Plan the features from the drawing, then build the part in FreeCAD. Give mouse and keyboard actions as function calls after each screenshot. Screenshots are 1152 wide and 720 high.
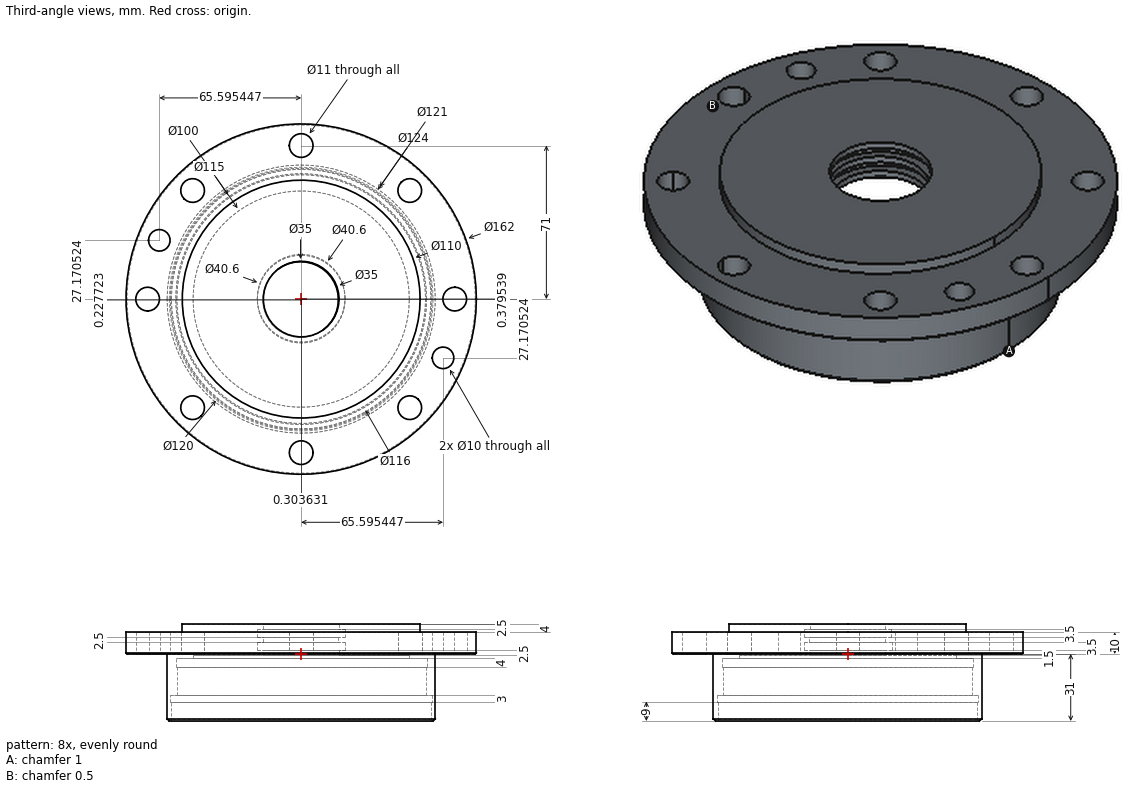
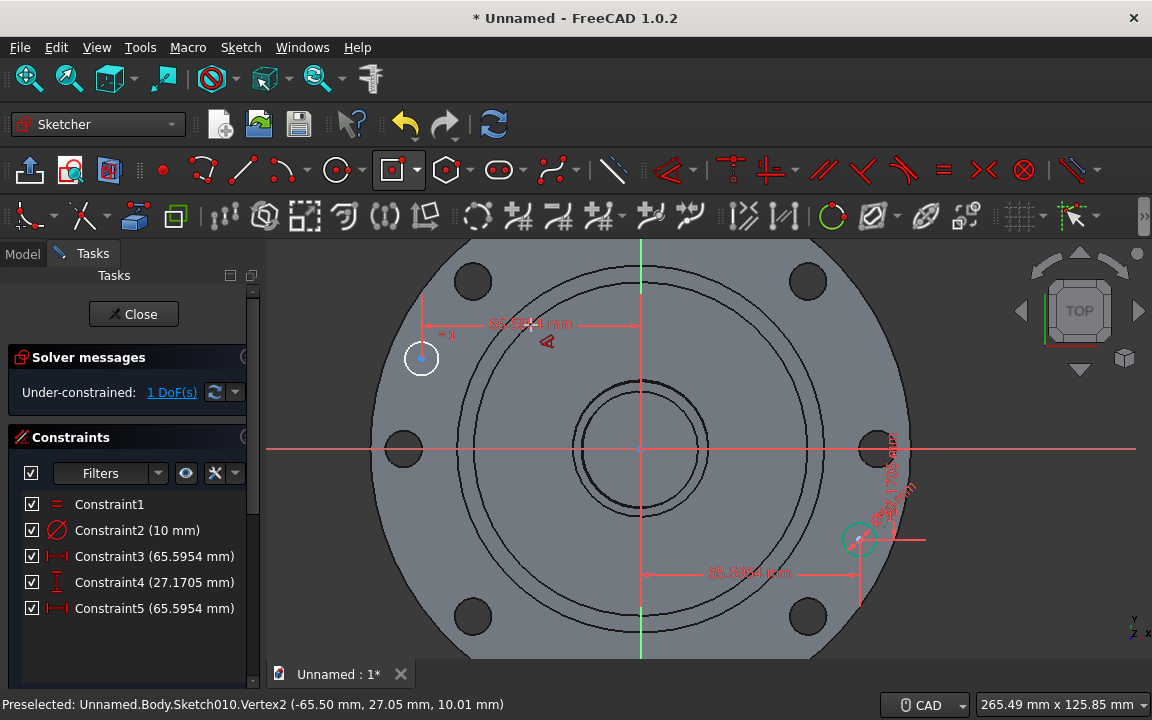
click(422, 359)
click(388, 404)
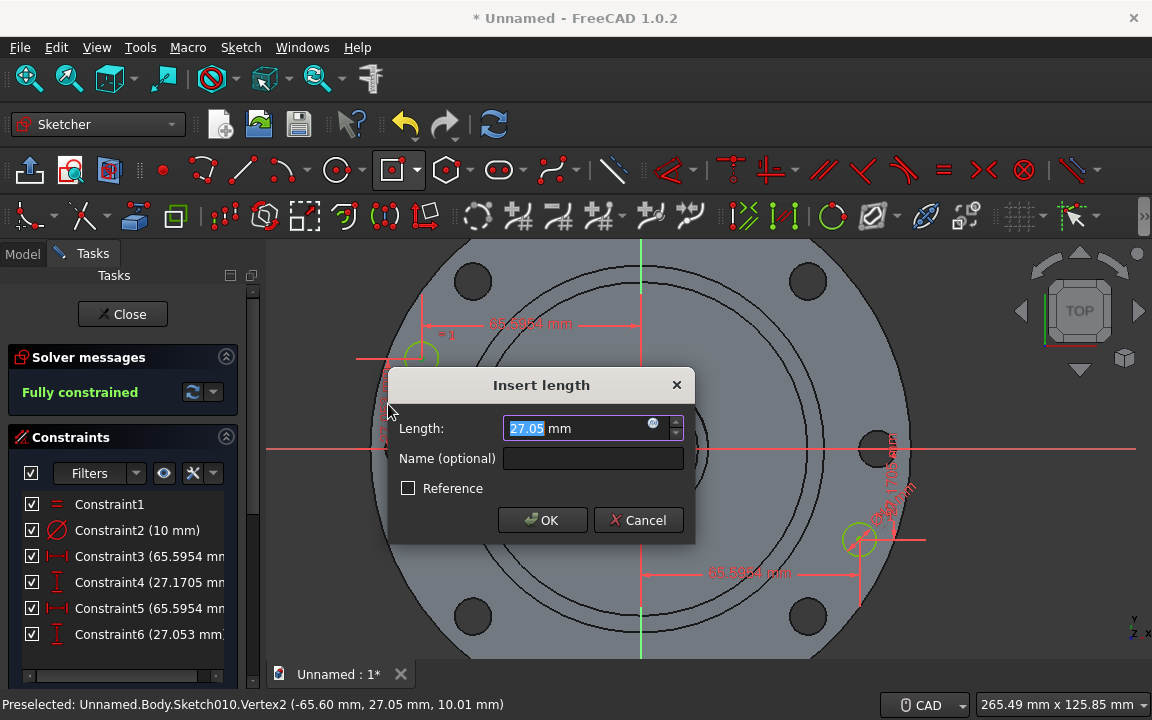
text(27.170524)
key(Return)
key(Escape)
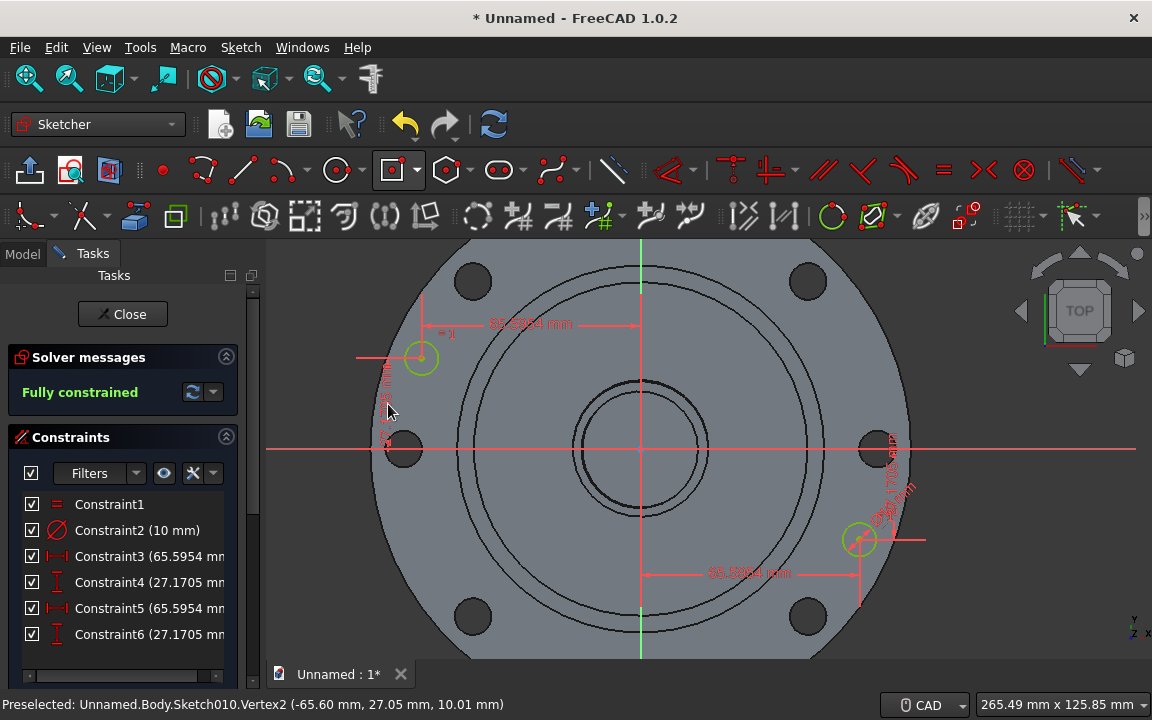
click(123, 314)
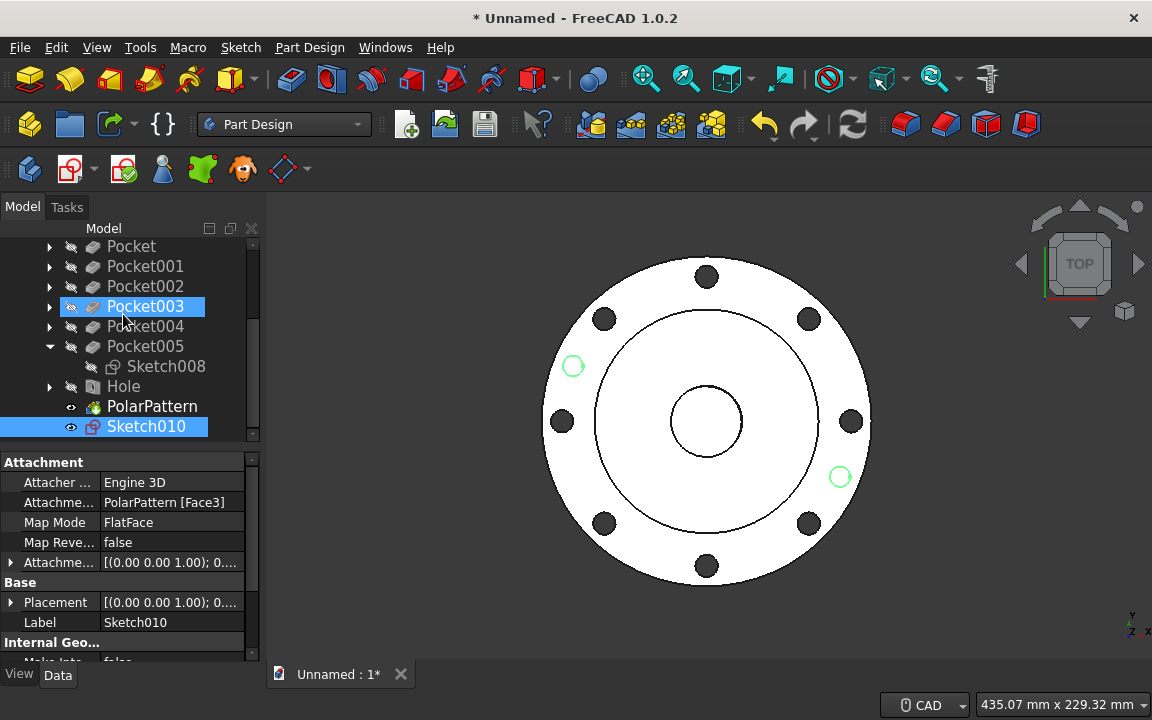
click(332, 80)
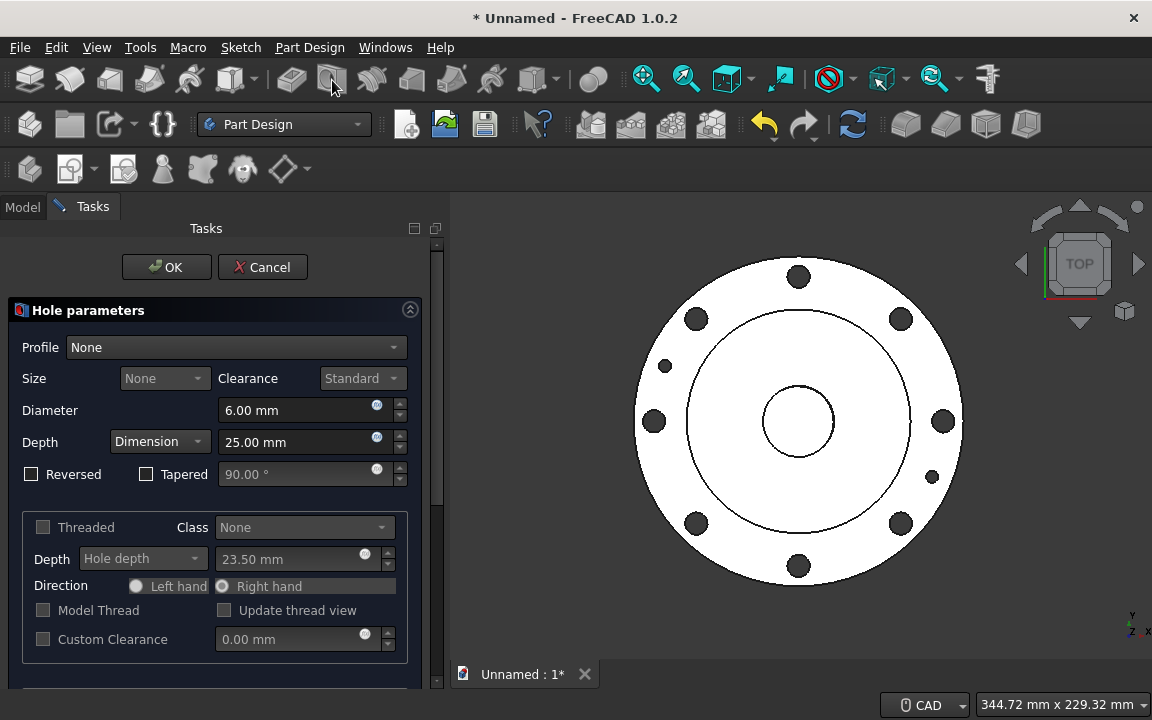
triple_click(305, 410)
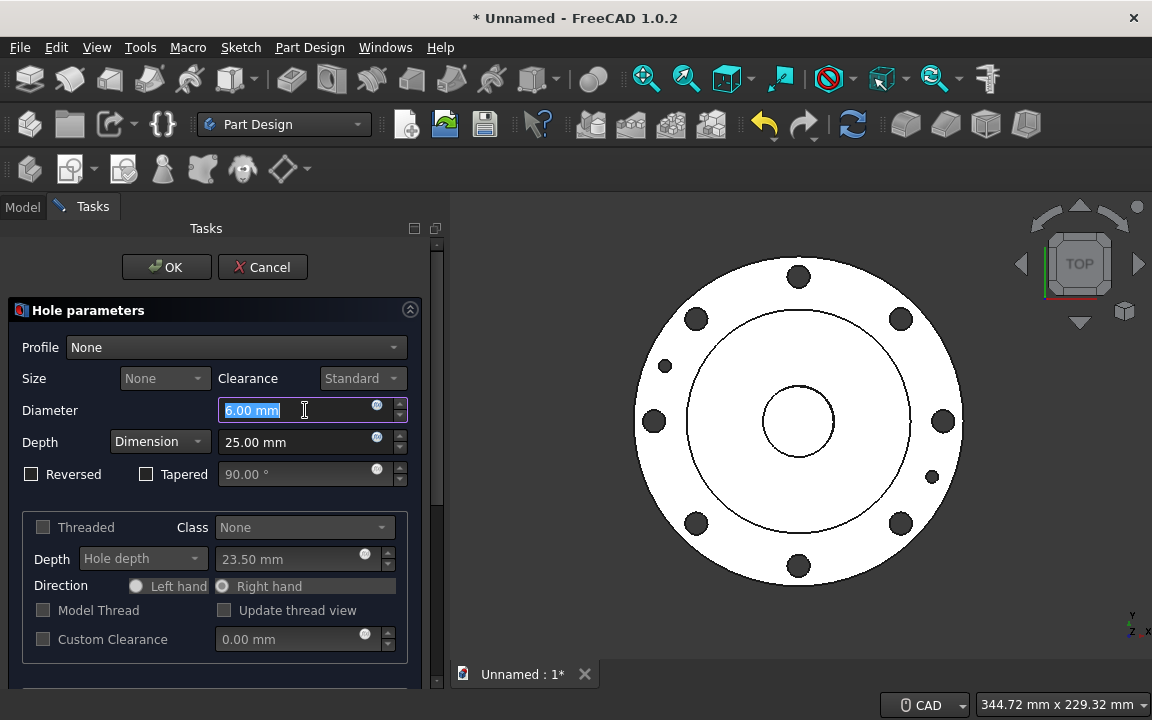
text(10)
key(Tab)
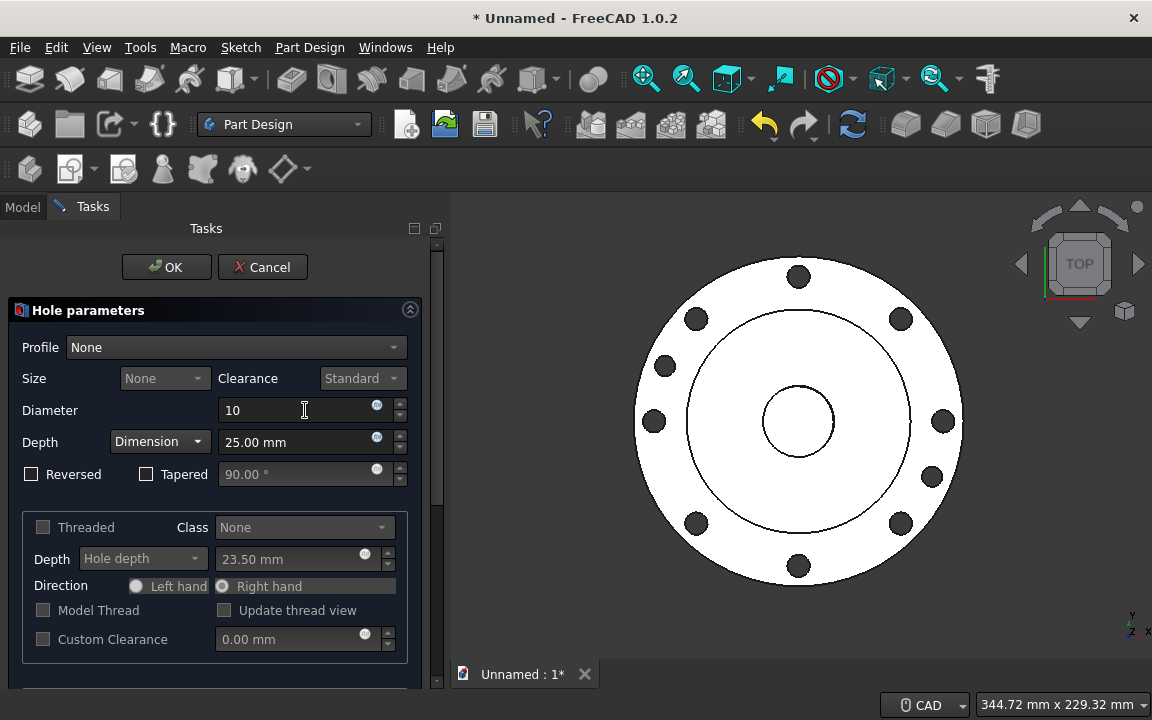
click(161, 442)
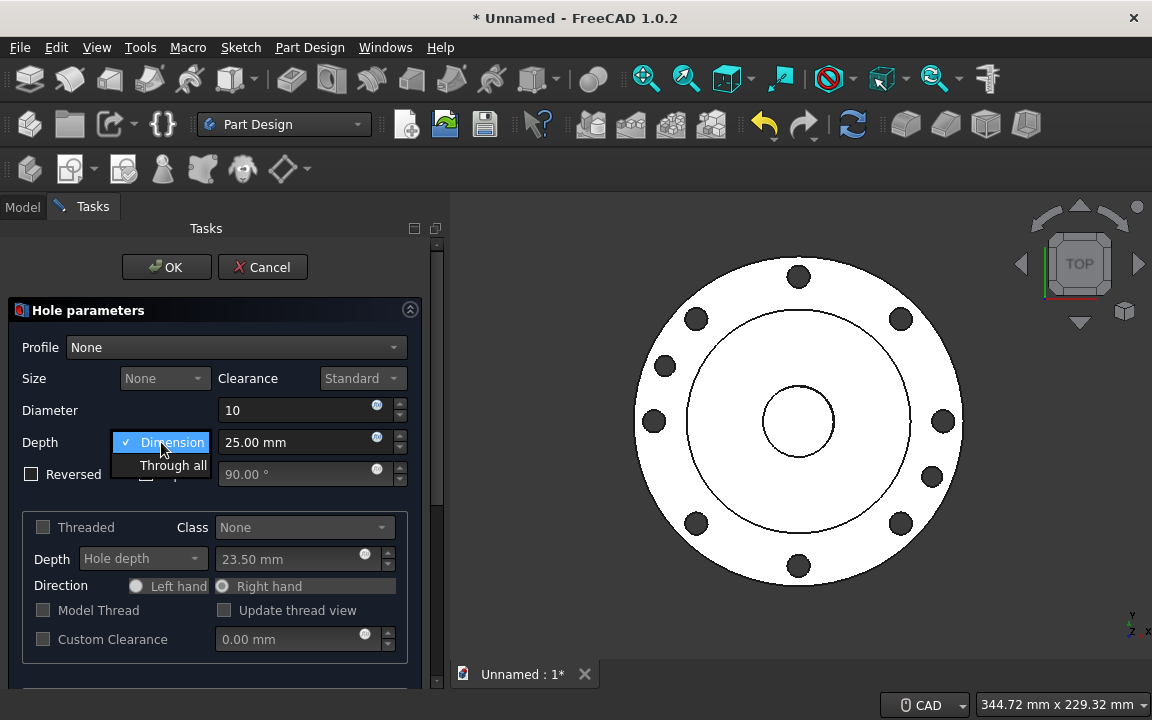
click(160, 466)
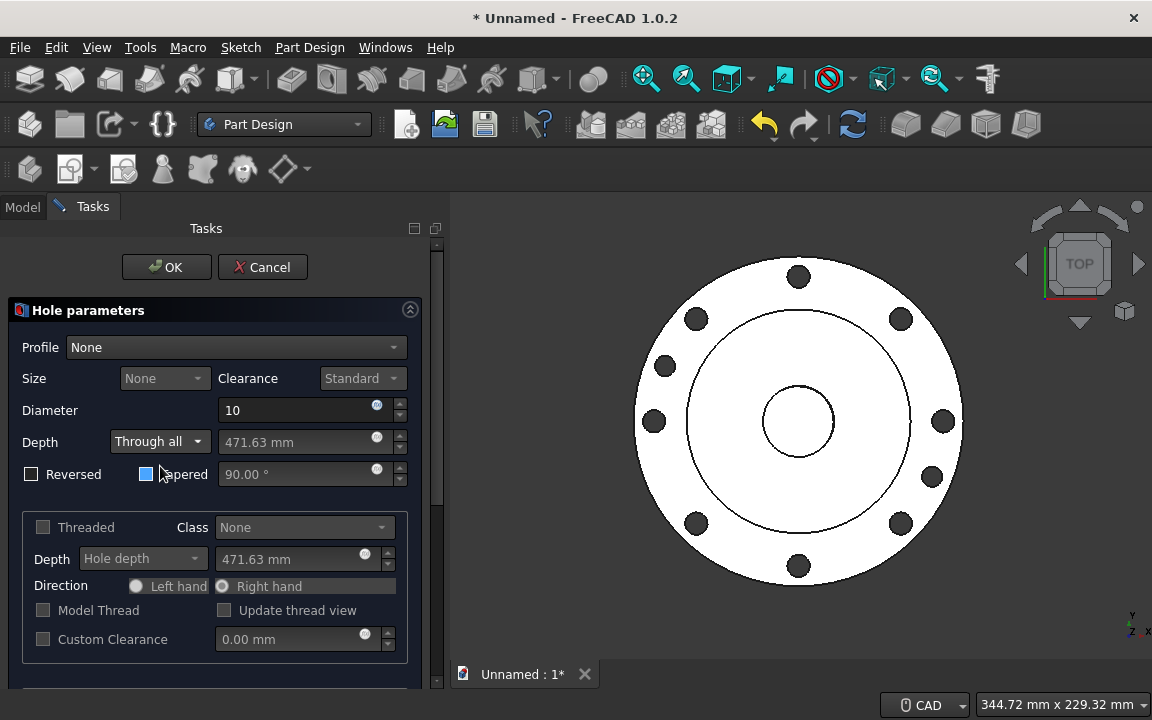
click(167, 267)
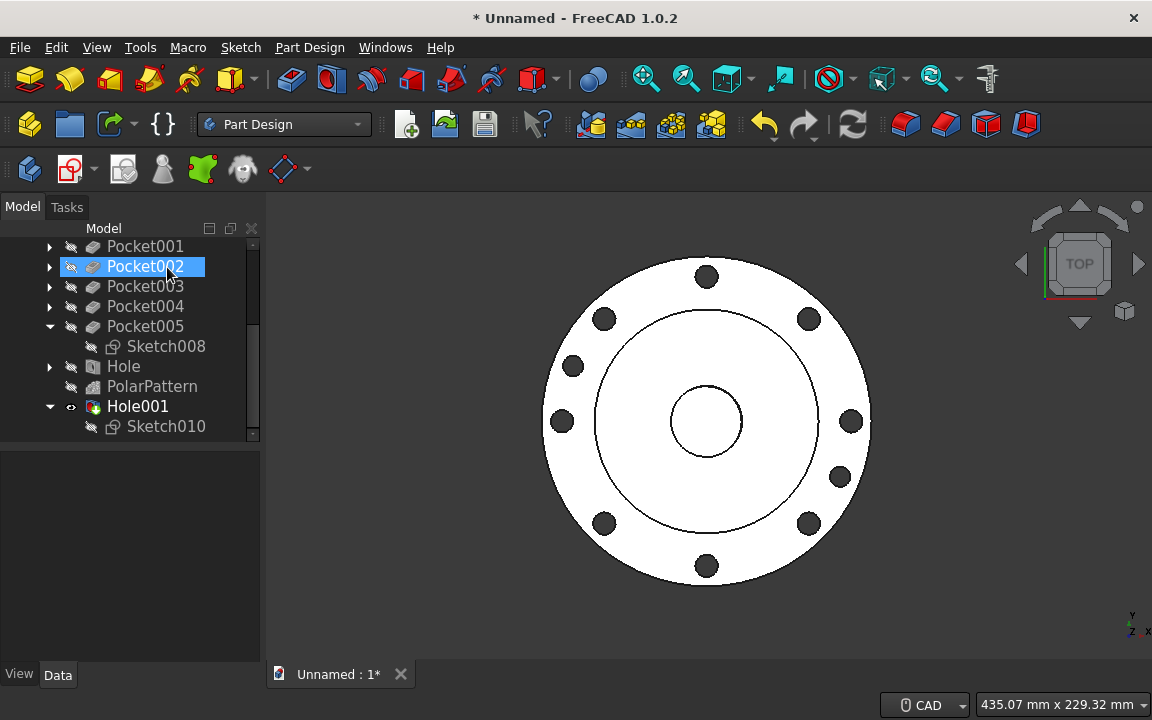
click(707, 420)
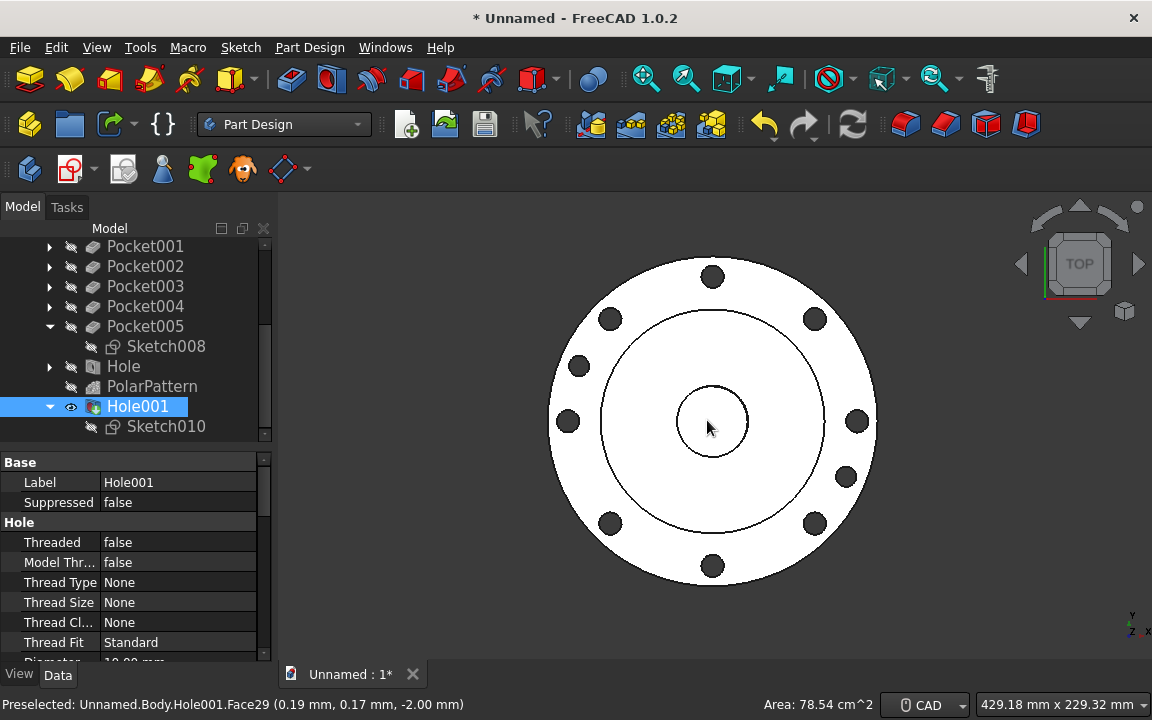
click(70, 170)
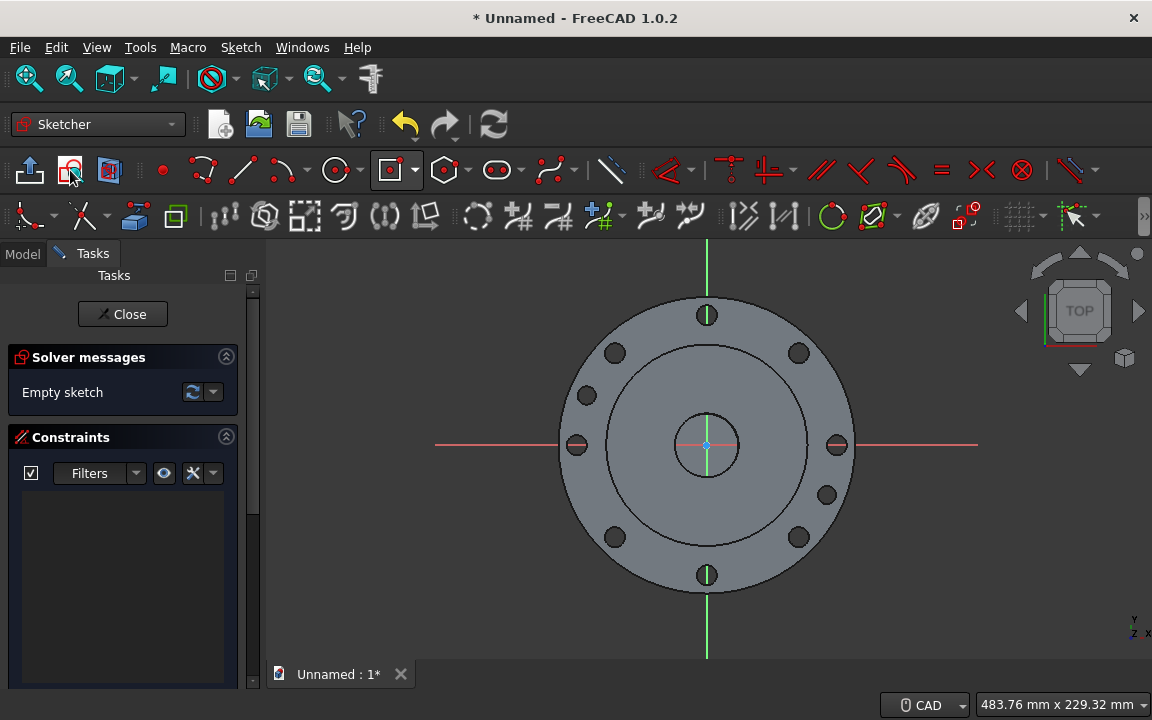
click(336, 170)